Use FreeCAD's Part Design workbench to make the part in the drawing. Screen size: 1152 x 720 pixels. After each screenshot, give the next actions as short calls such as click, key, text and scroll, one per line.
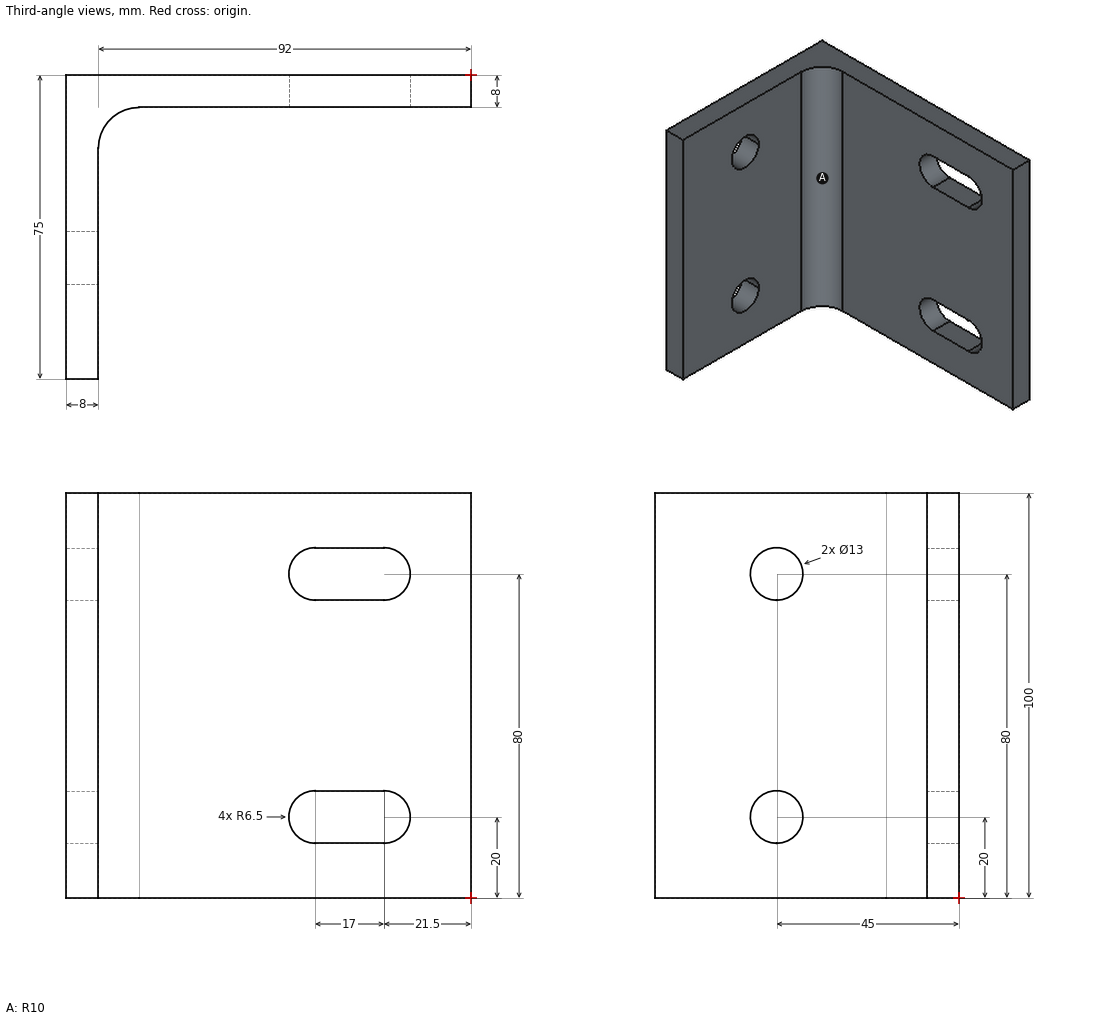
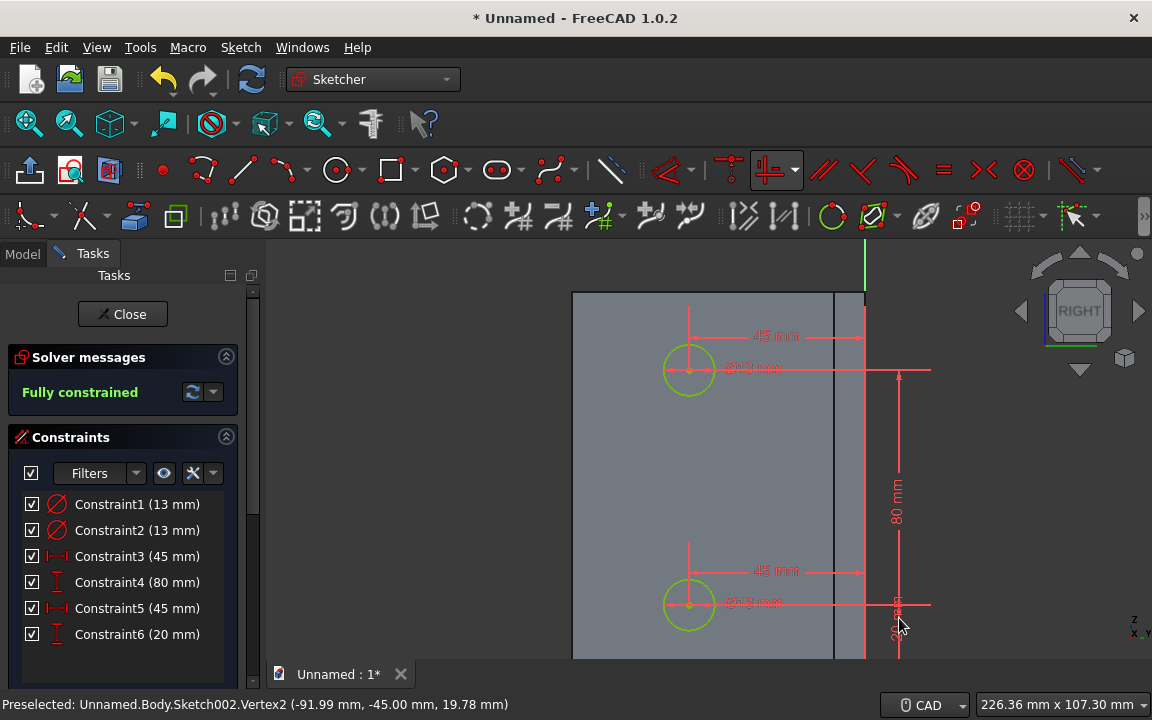
click(123, 314)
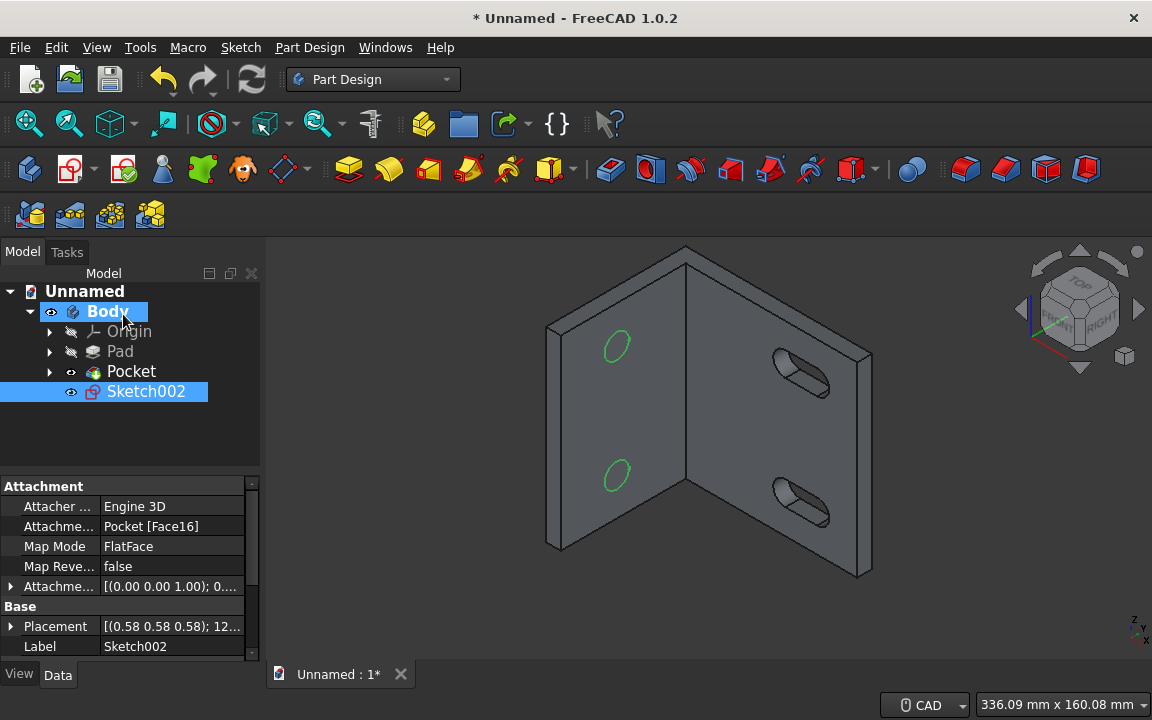
click(612, 170)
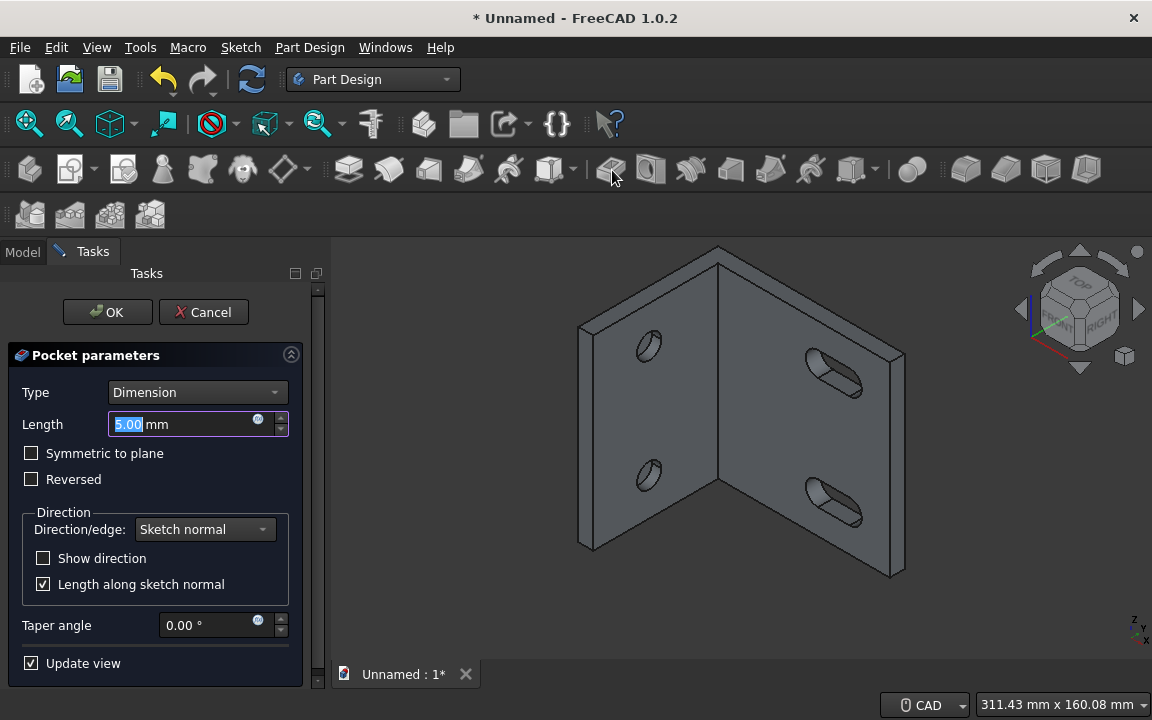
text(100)
key(Tab)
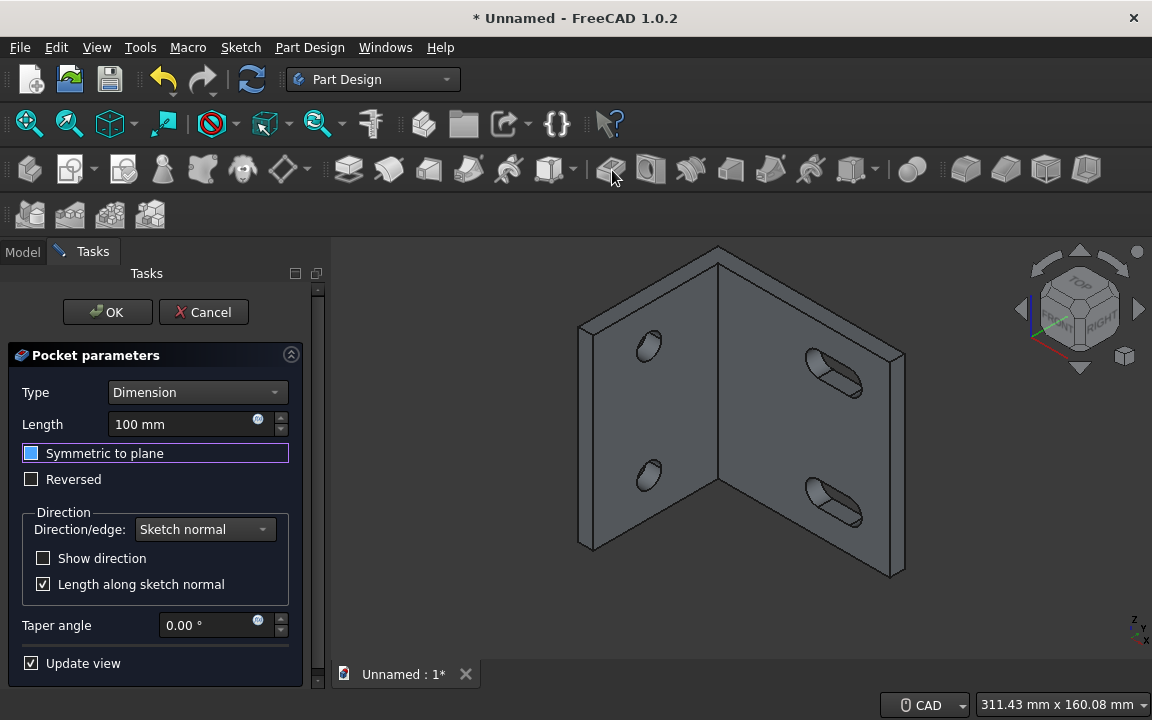
click(108, 312)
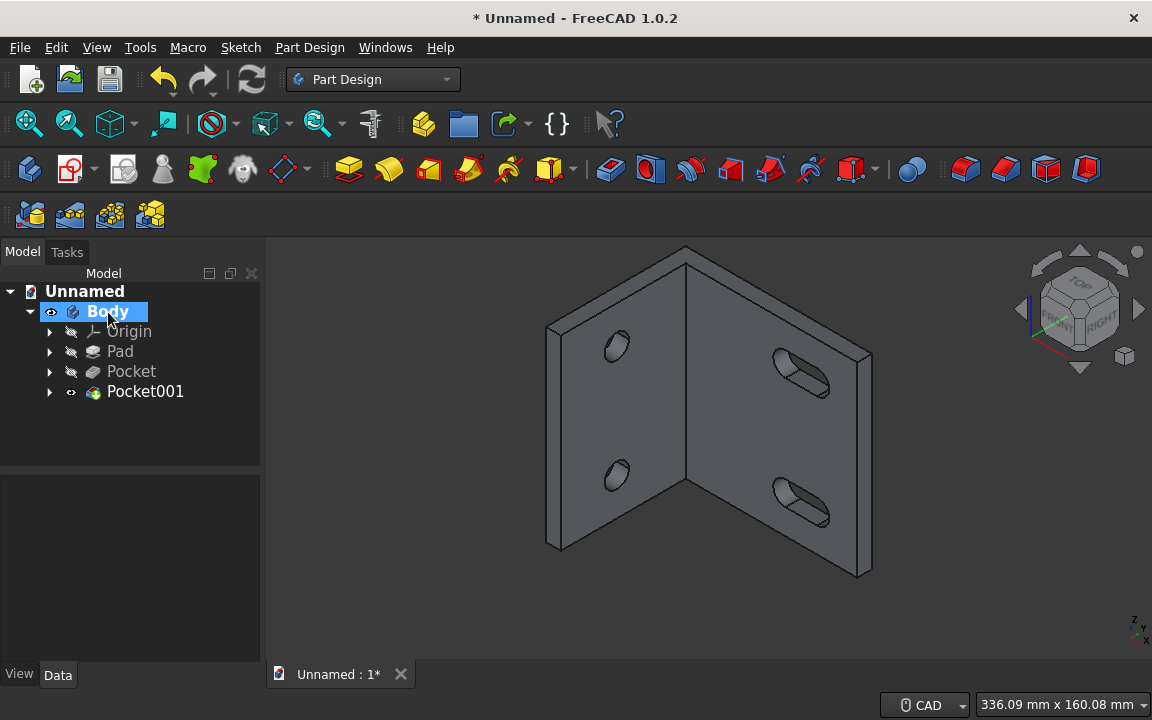
key(2)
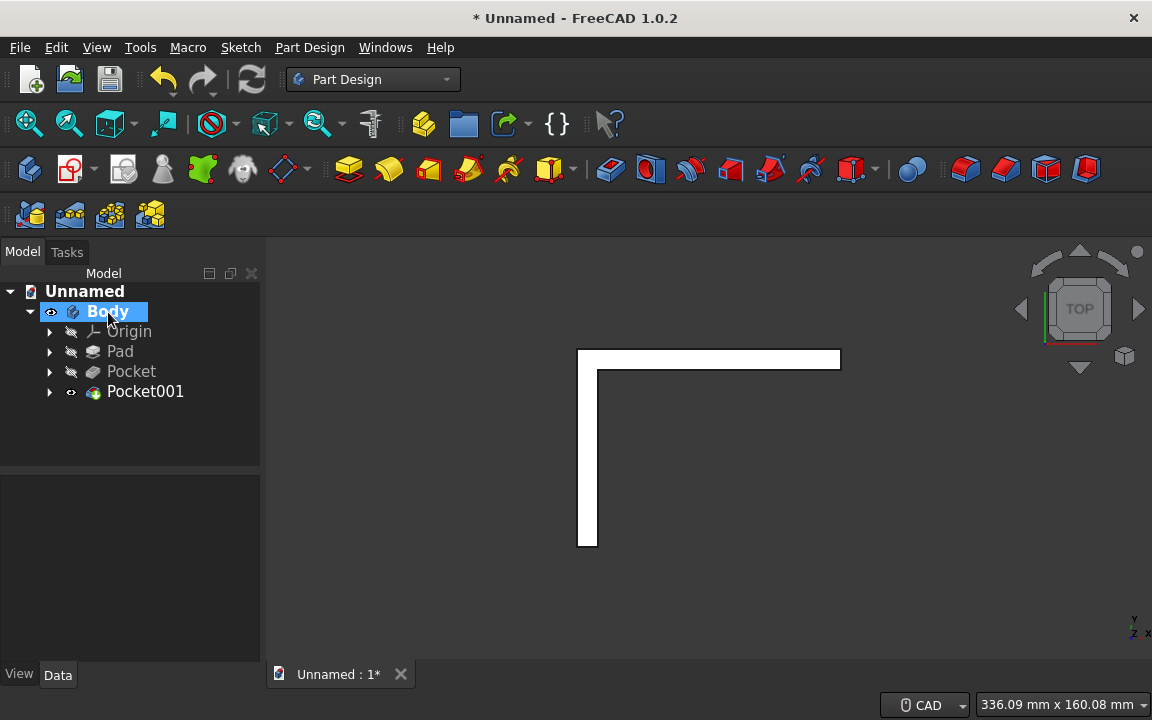
key(0)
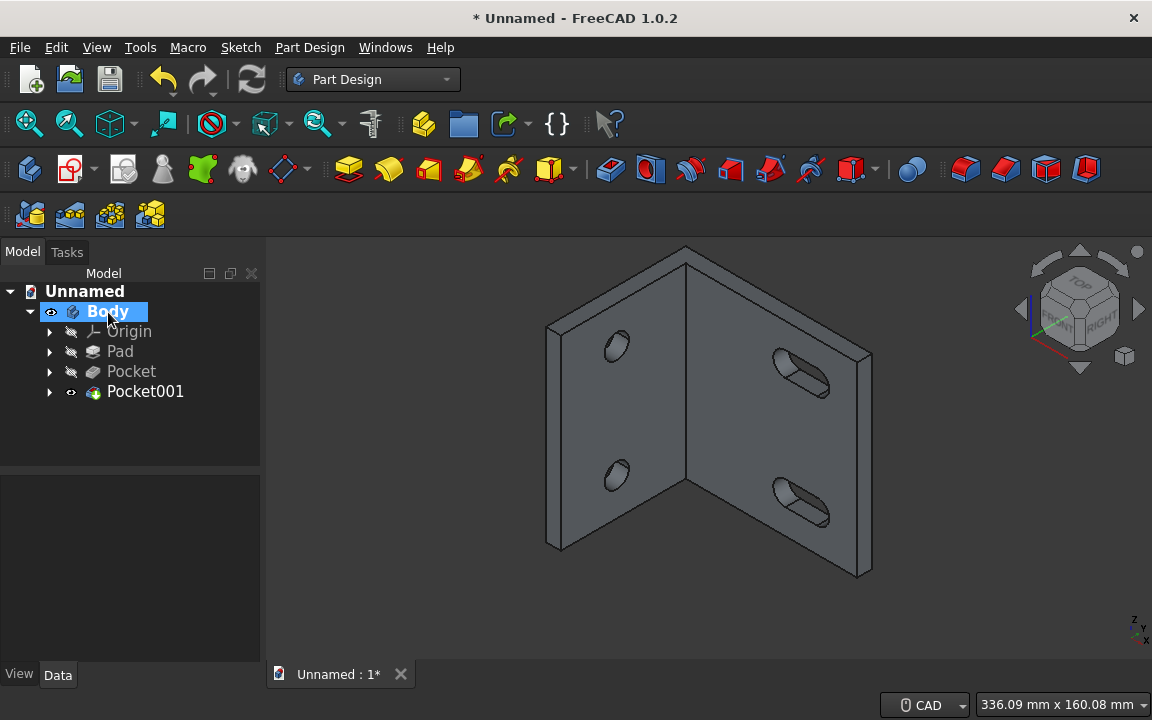
key(1)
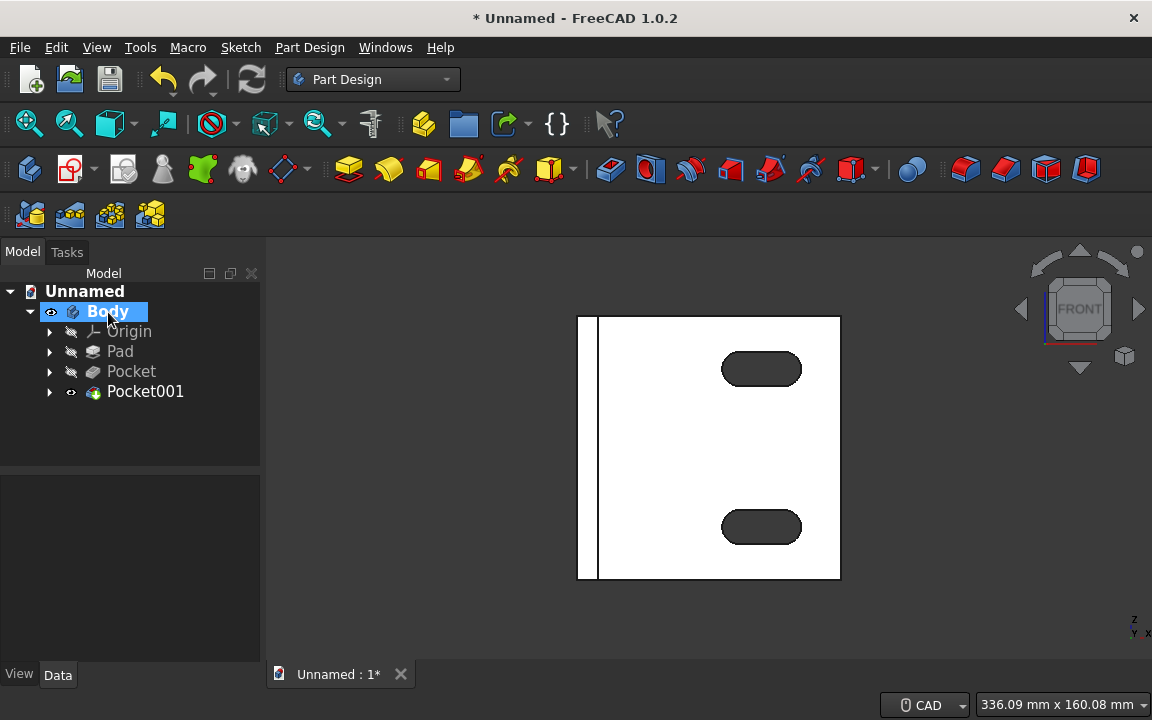
key(3)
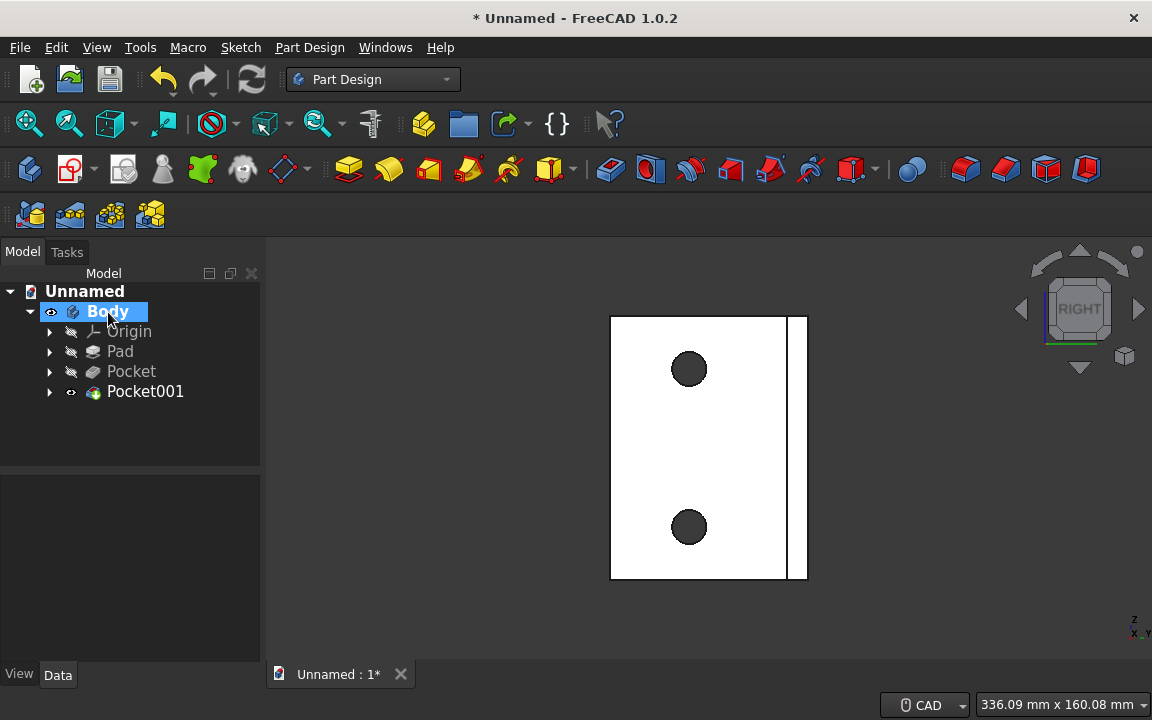
key(5)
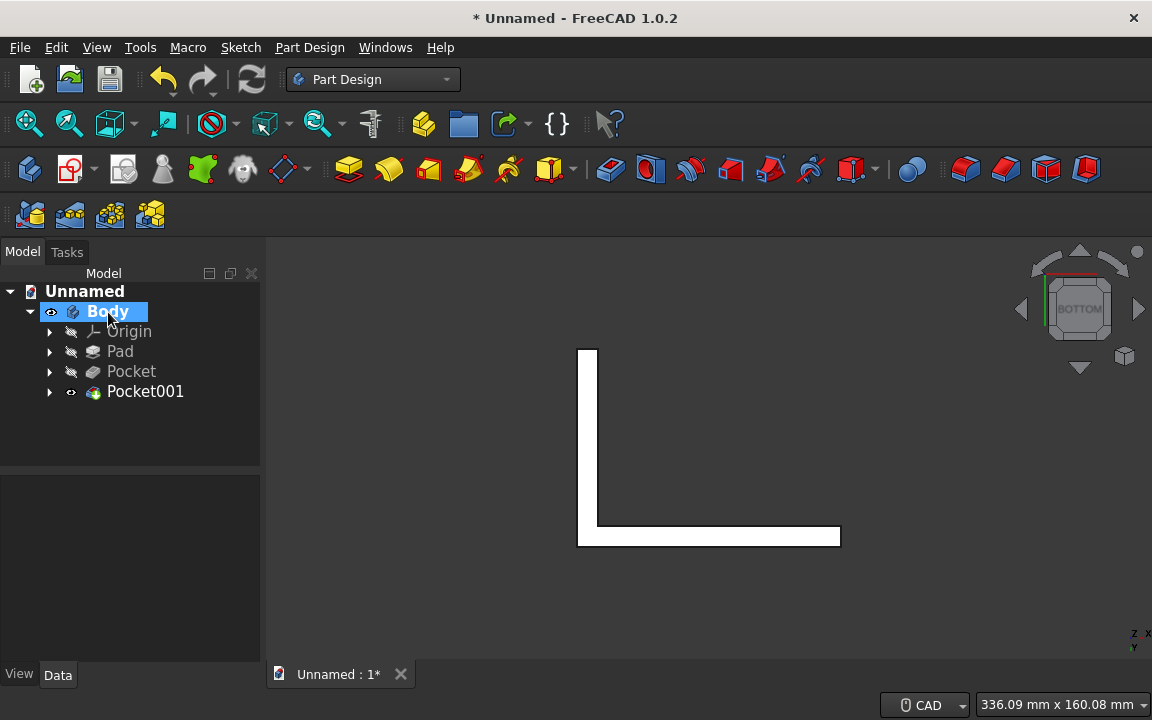
key(4)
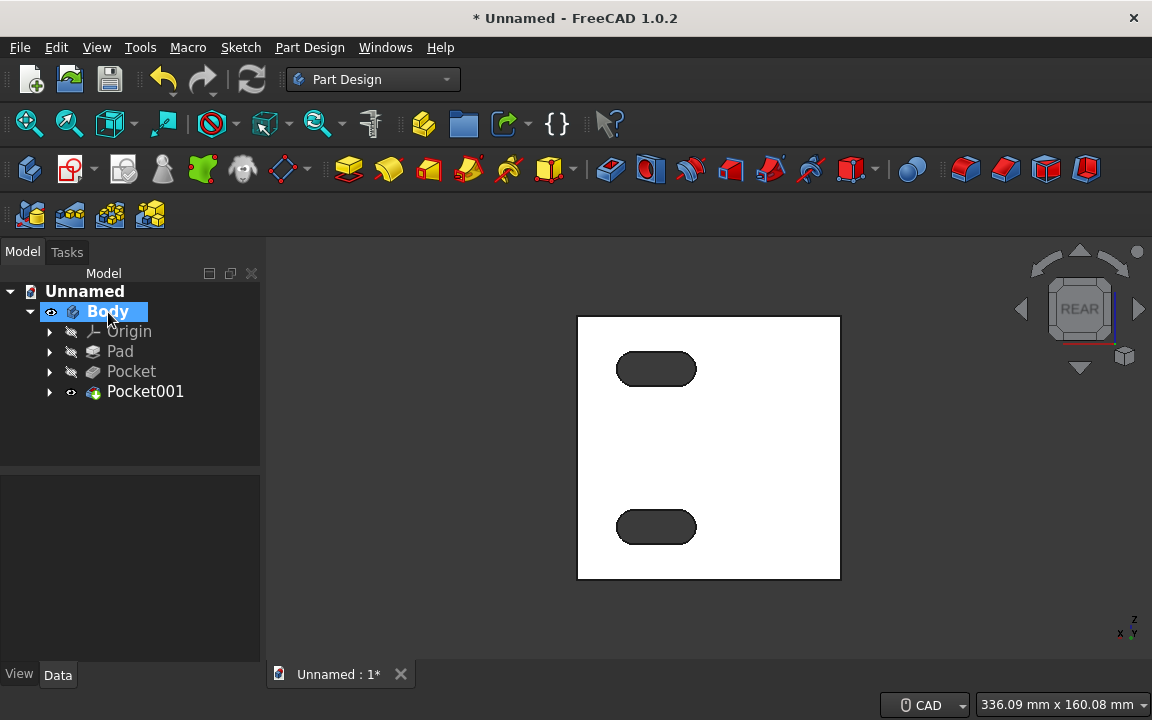
key(6)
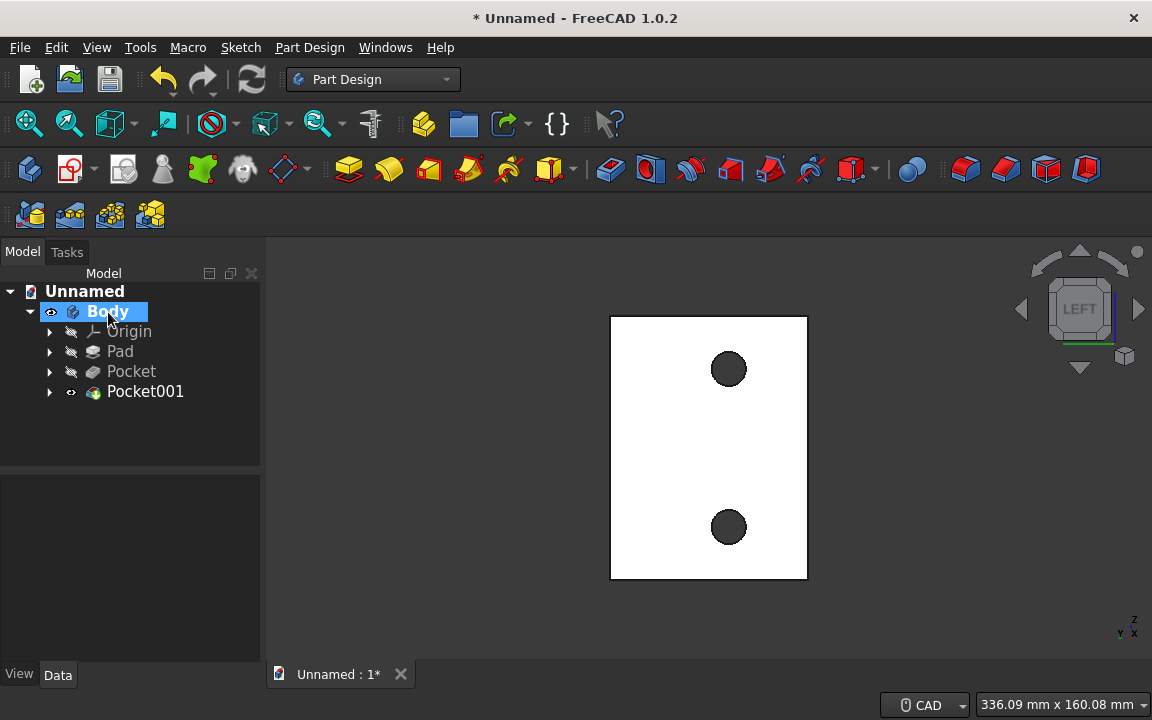
key(v)
key(3)